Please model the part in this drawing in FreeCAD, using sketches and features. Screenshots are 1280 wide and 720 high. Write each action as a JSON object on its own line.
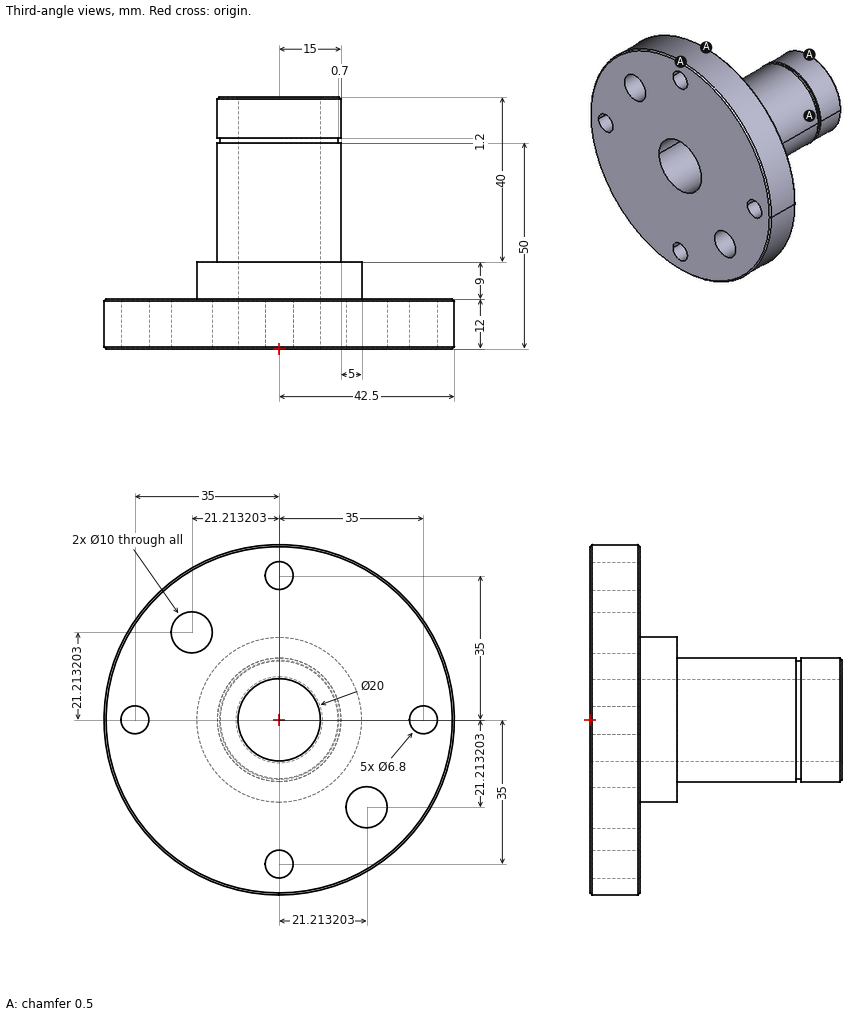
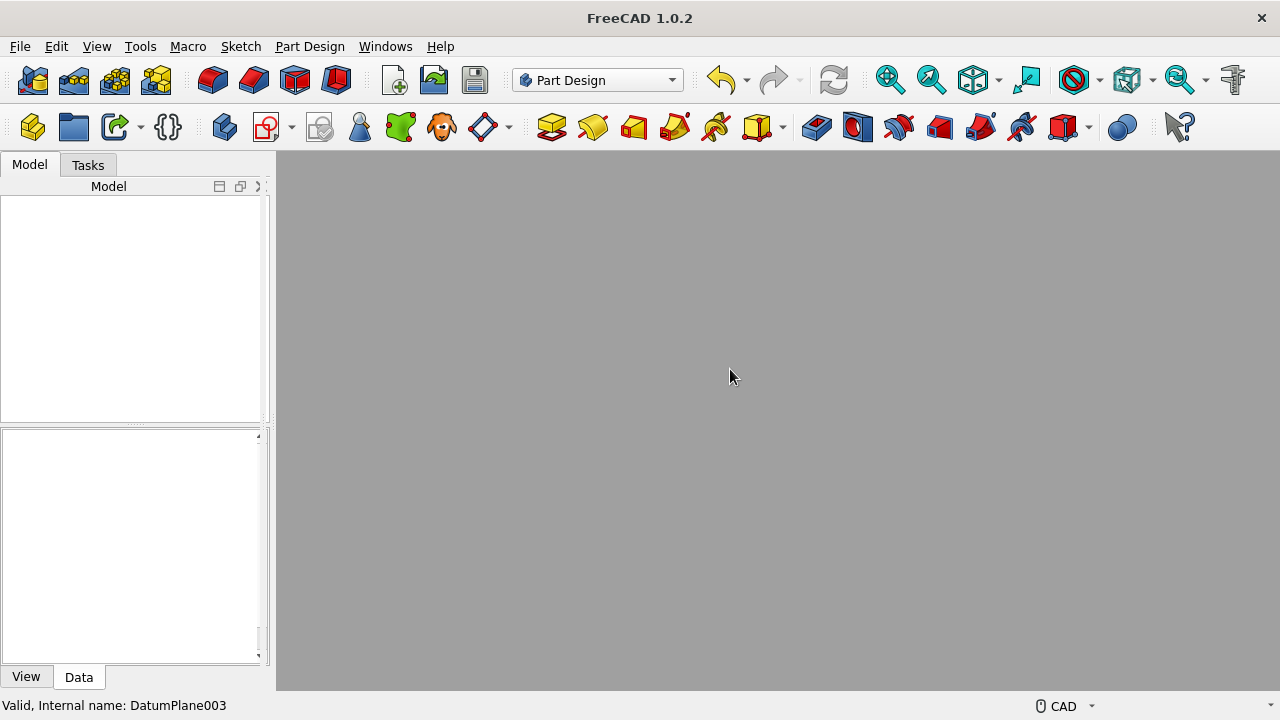
{"action": "key", "text": "ctrl+n"}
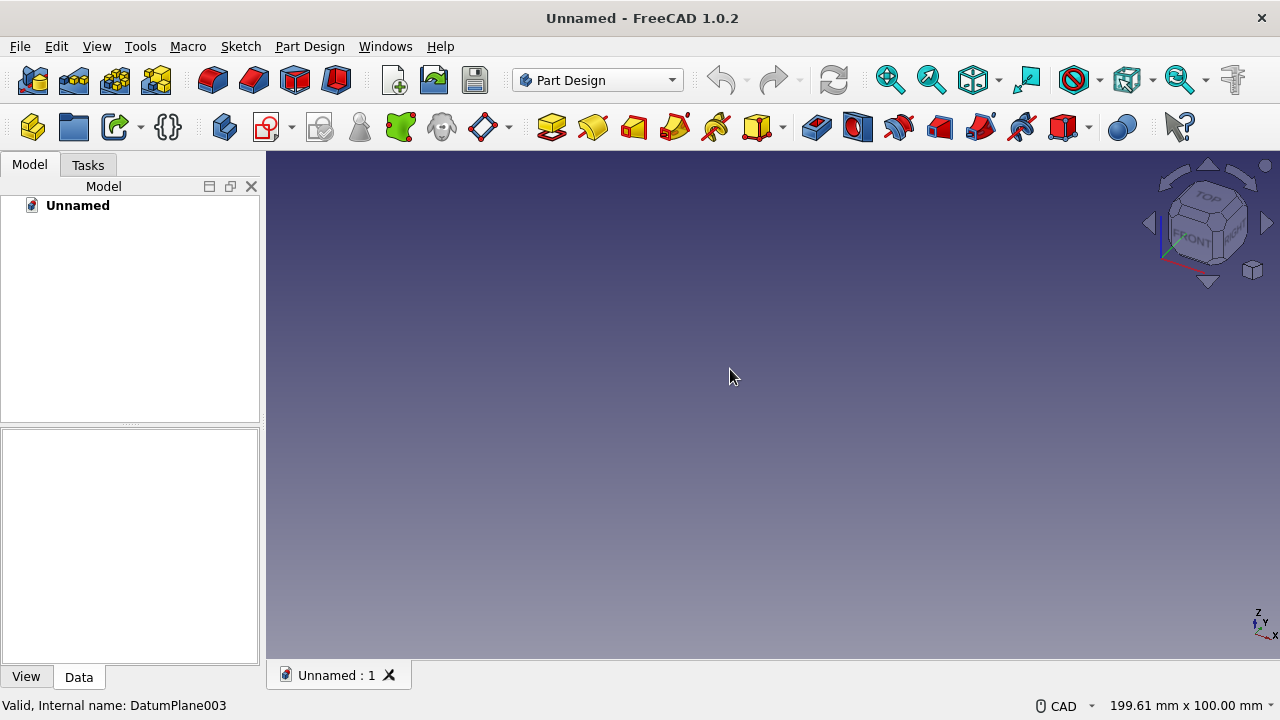
{"action": "left_click", "coordinate": [266, 128]}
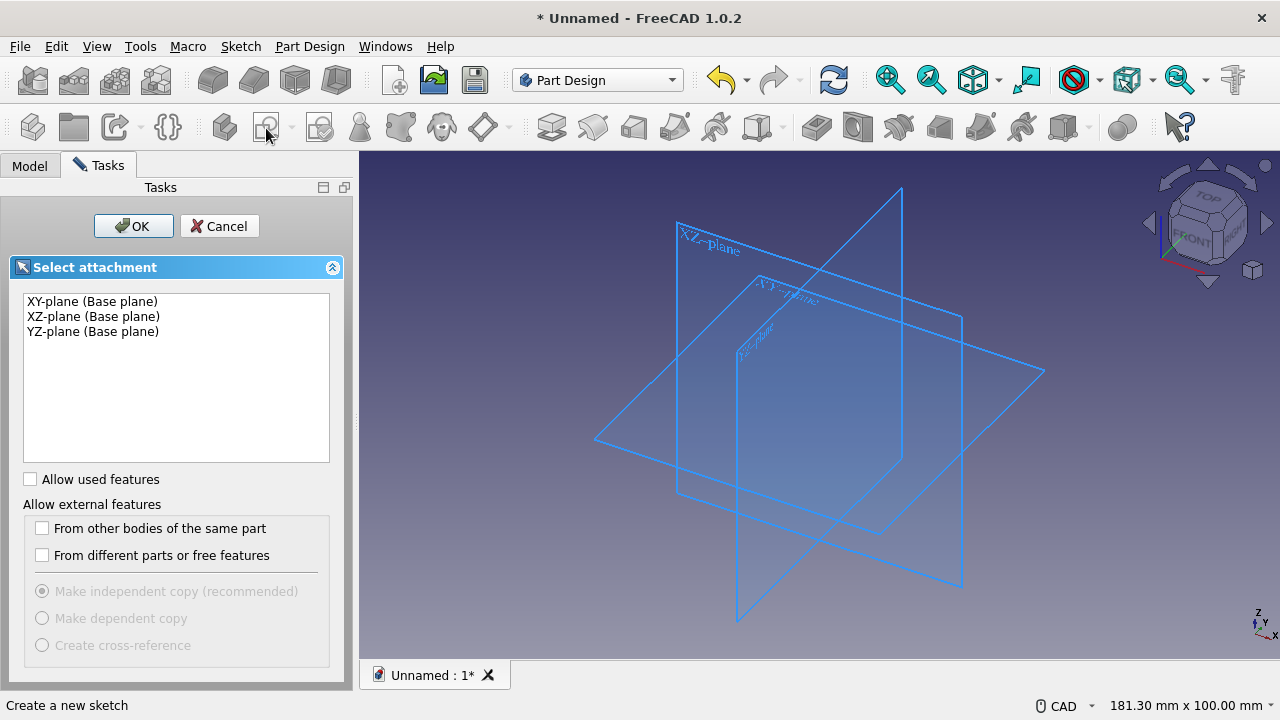
{"action": "left_click", "coordinate": [84, 302]}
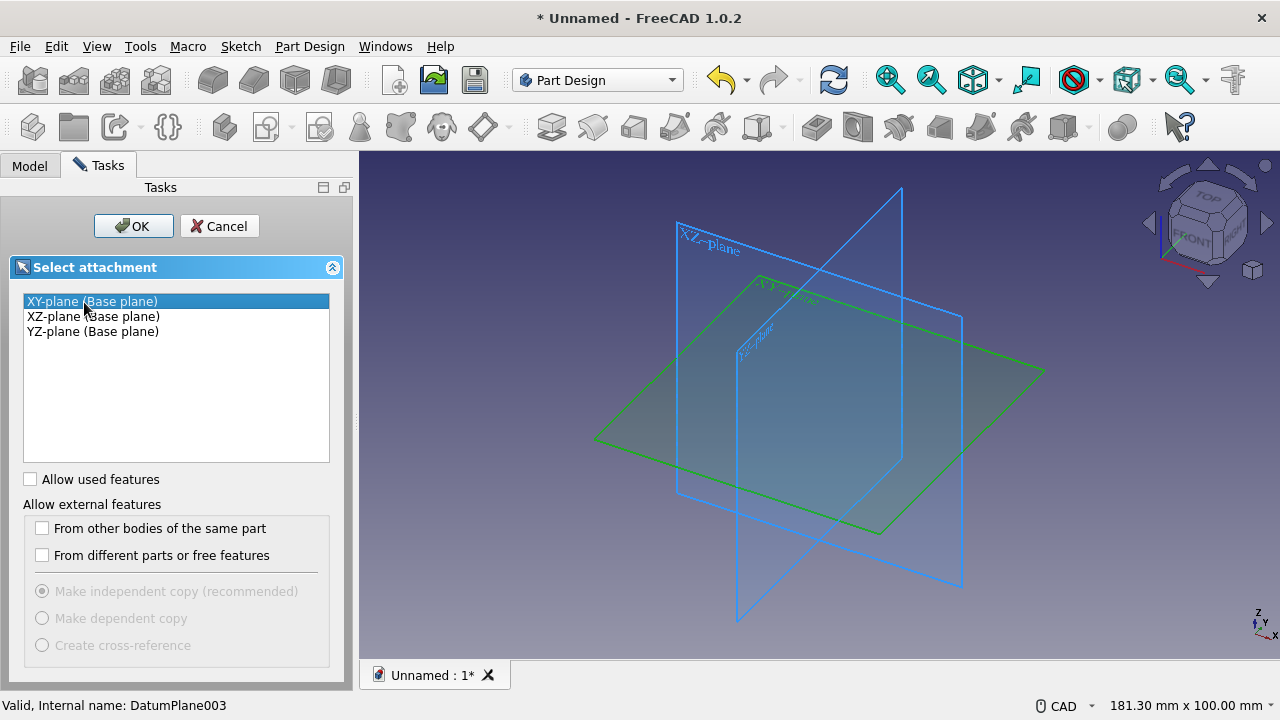
{"action": "left_click", "coordinate": [134, 226]}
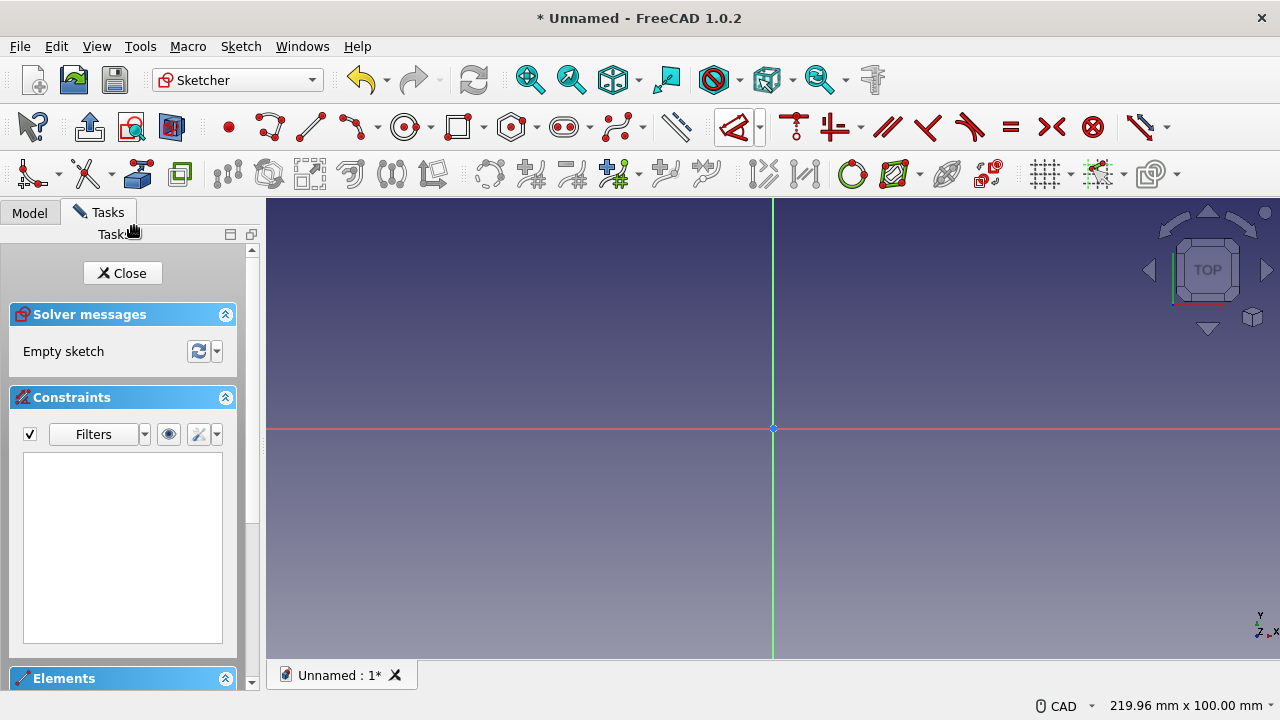
{"action": "scroll", "coordinate": [366, 631], "scroll_direction": "down", "scroll_amount": 2}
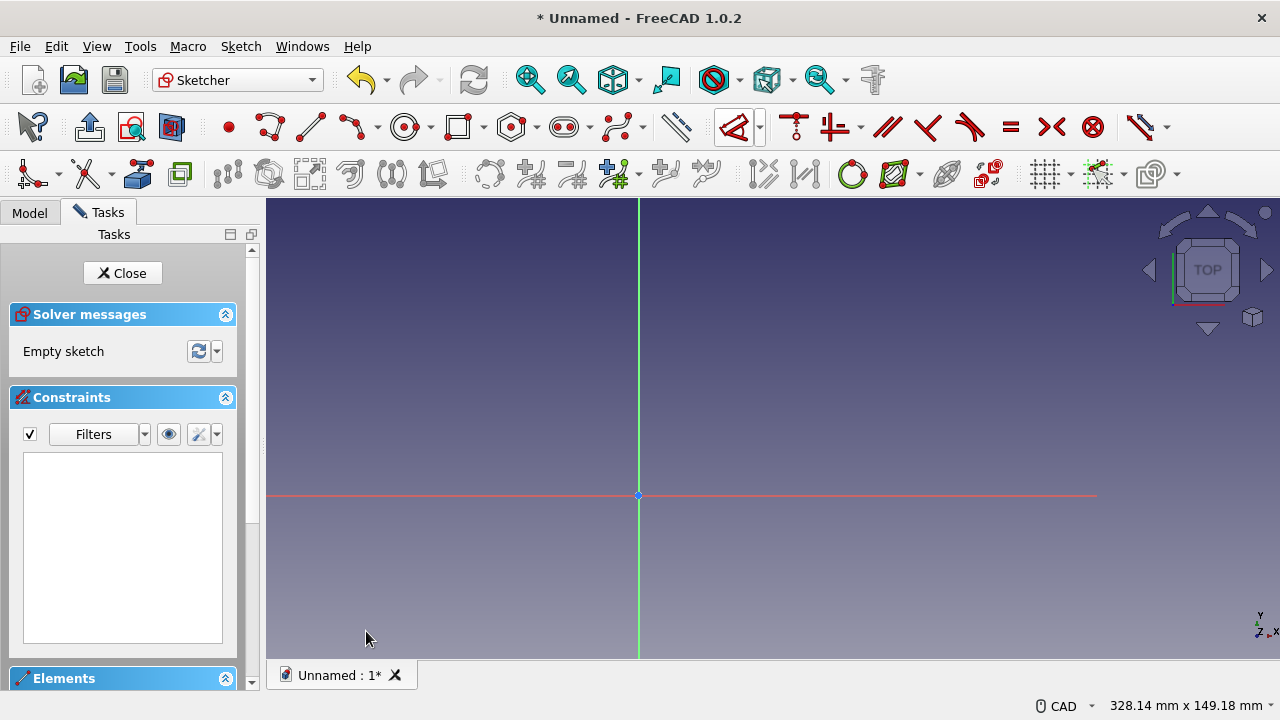
{"action": "scroll", "coordinate": [705, 346], "scroll_direction": "up", "scroll_amount": 2}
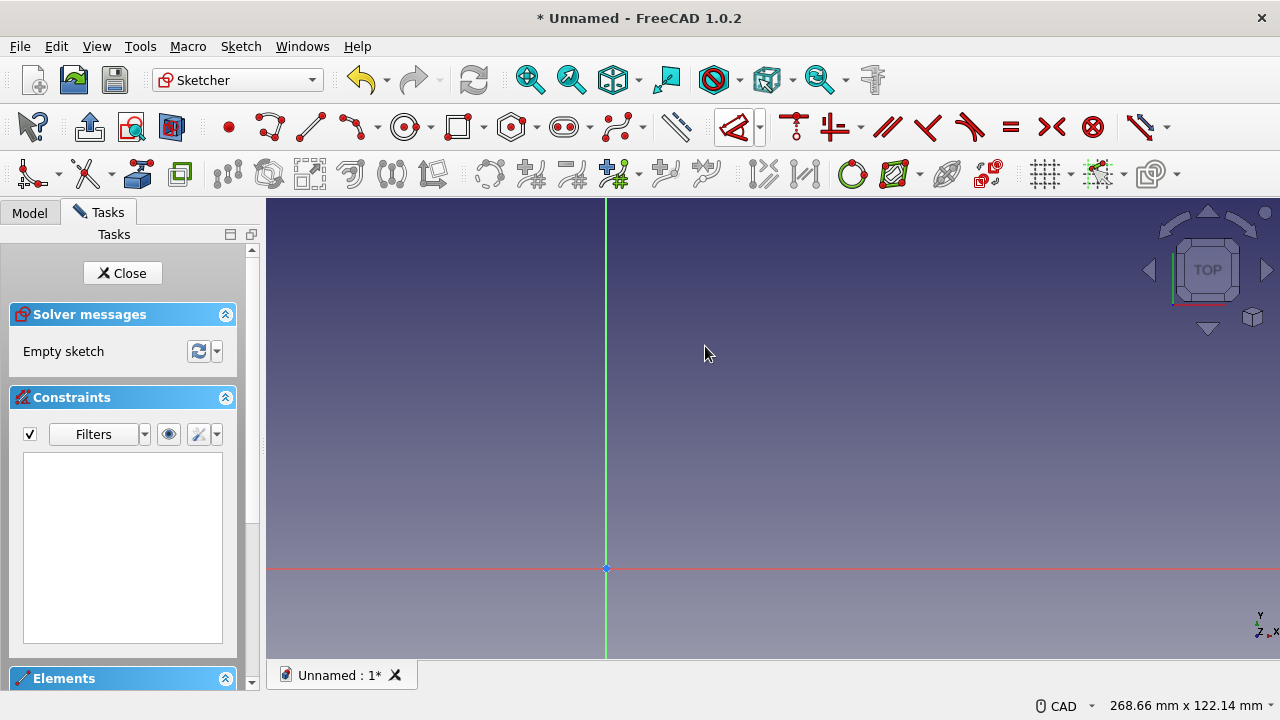
{"action": "key", "text": "g m"}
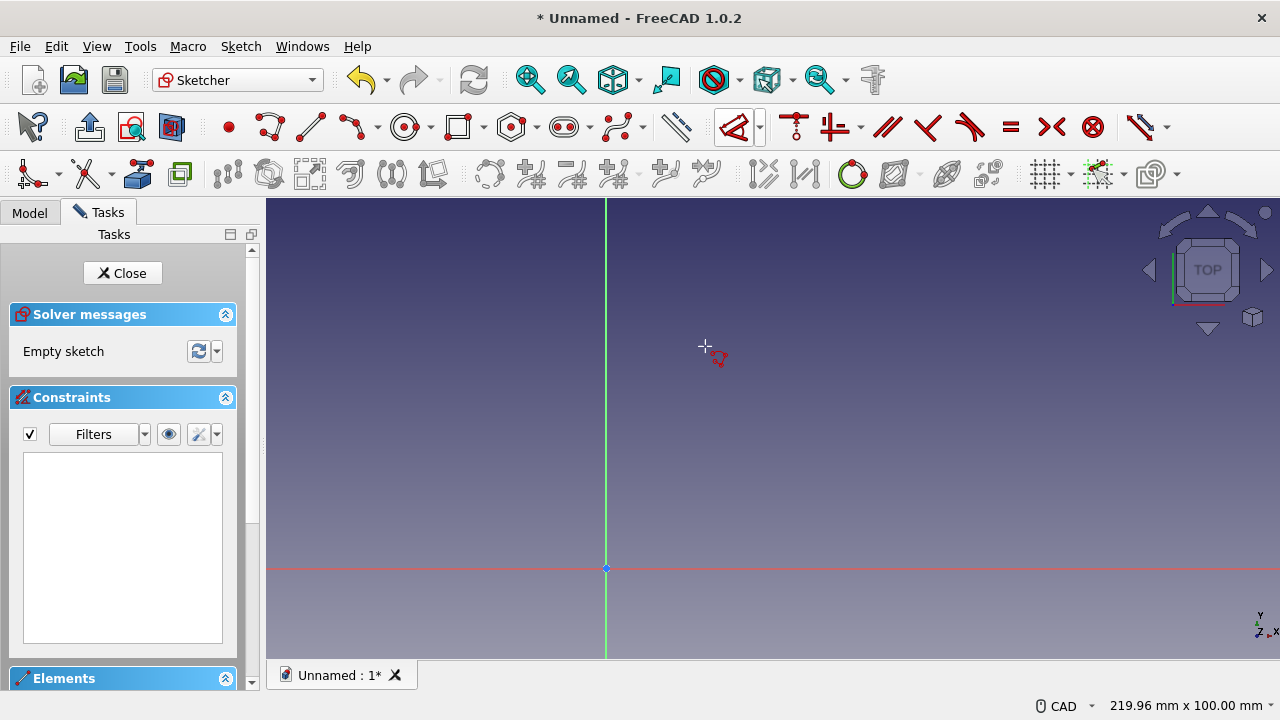
{"action": "left_click", "coordinate": [606, 569]}
{"action": "left_click", "coordinate": [802, 560]}
{"action": "left_click", "coordinate": [802, 514]}
{"action": "left_click", "coordinate": [698, 514]}
{"action": "left_click", "coordinate": [698, 472]}
{"action": "left_click", "coordinate": [675, 472]}
{"action": "left_click", "coordinate": [675, 288]}
{"action": "left_click", "coordinate": [615, 288]}
{"action": "left_click", "coordinate": [606, 569]}
{"action": "key", "text": "Escape"}
{"action": "key", "text": "Escape"}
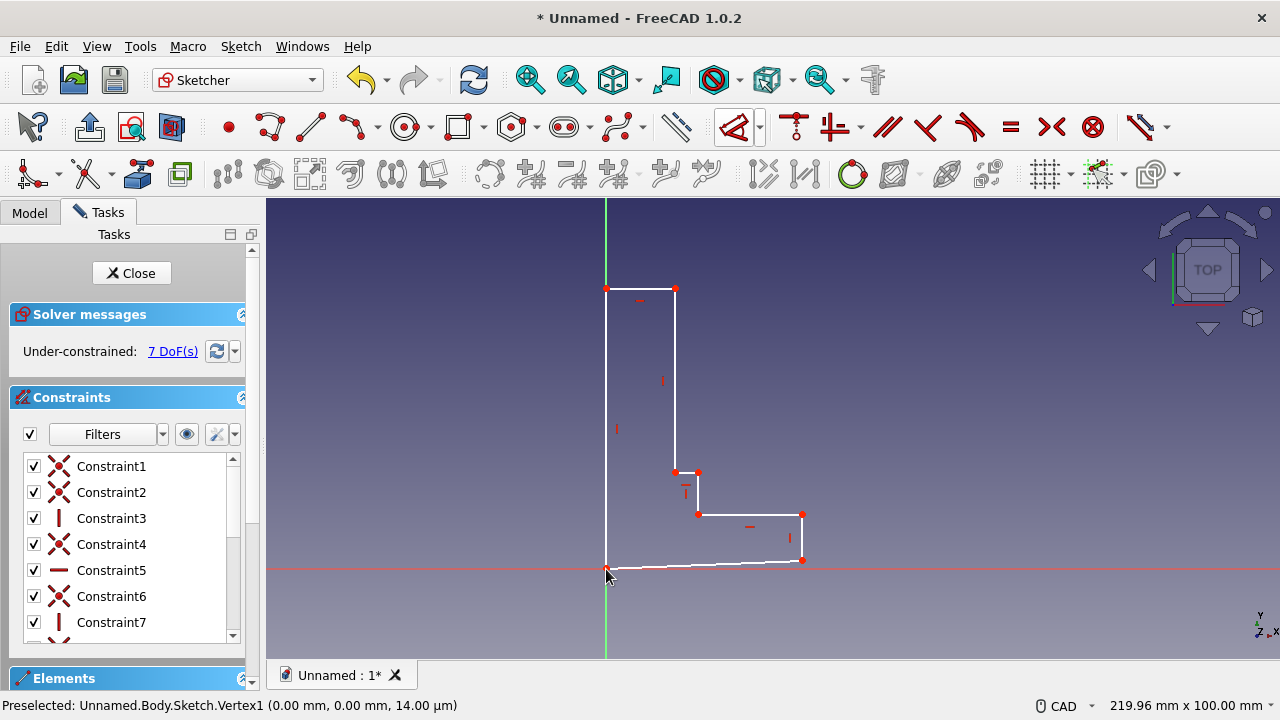
{"action": "left_click", "coordinate": [665, 567]}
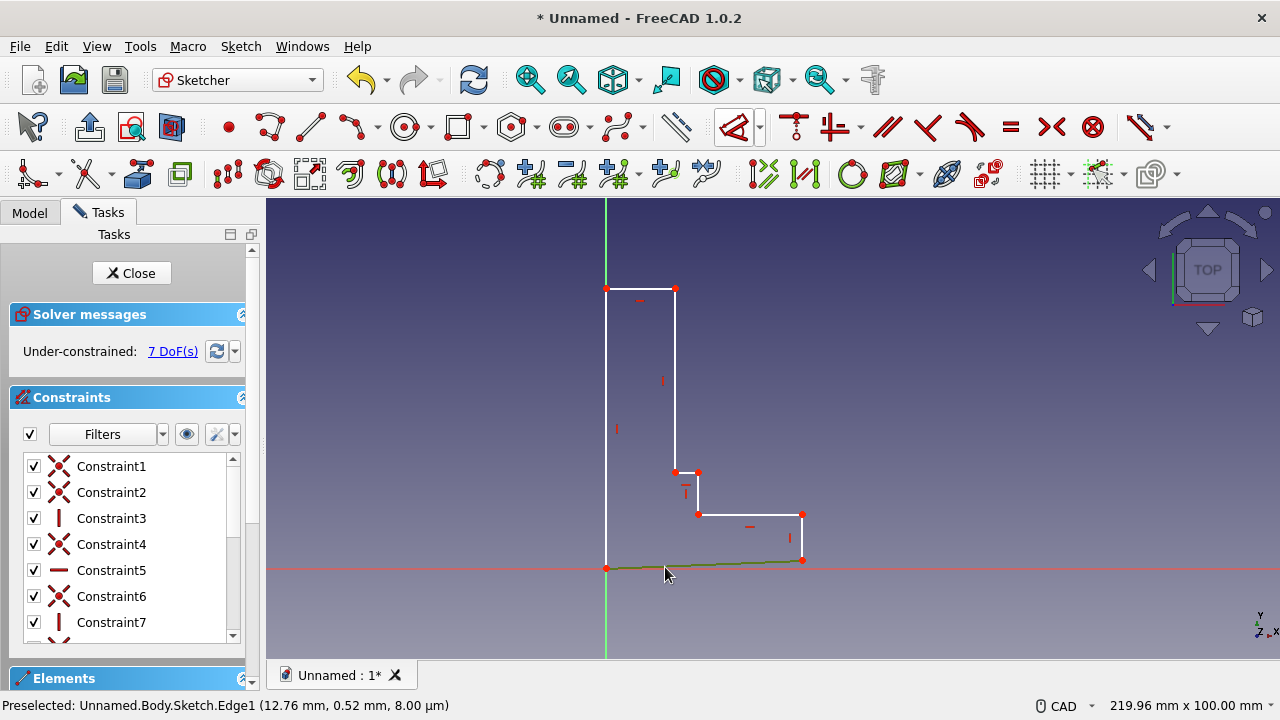
{"action": "key", "text": "h"}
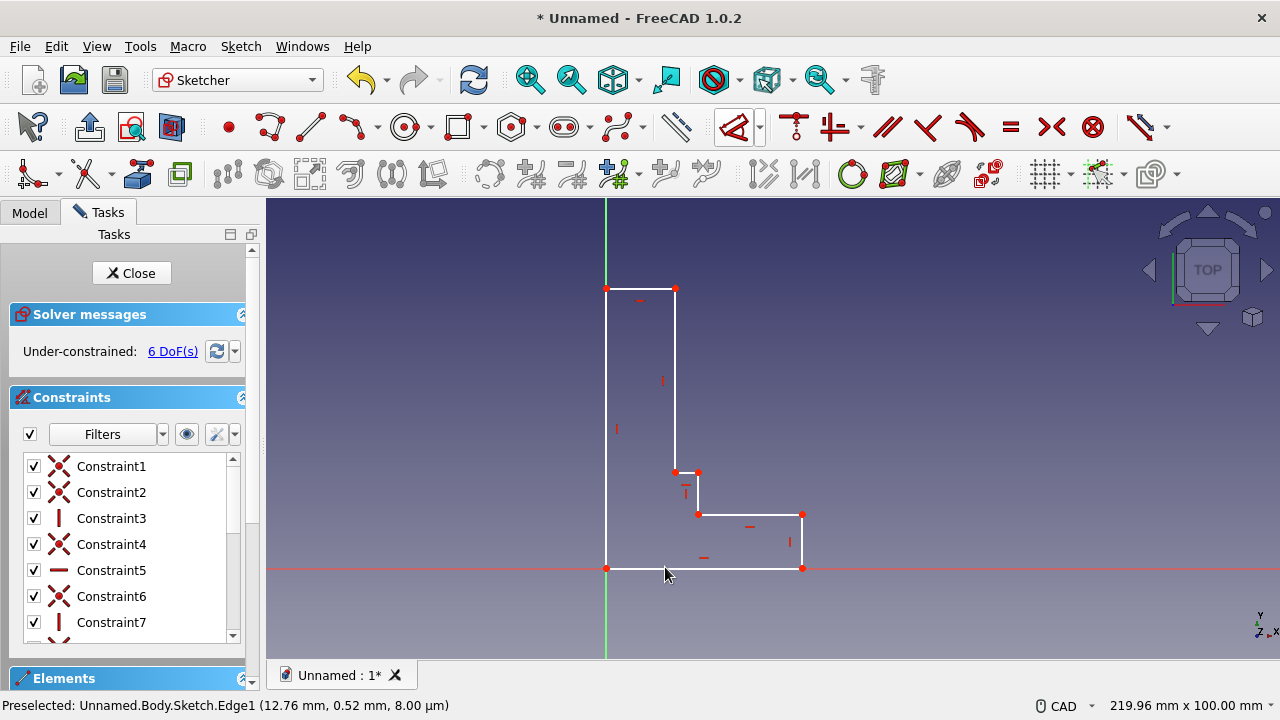
{"action": "left_click", "coordinate": [734, 128]}